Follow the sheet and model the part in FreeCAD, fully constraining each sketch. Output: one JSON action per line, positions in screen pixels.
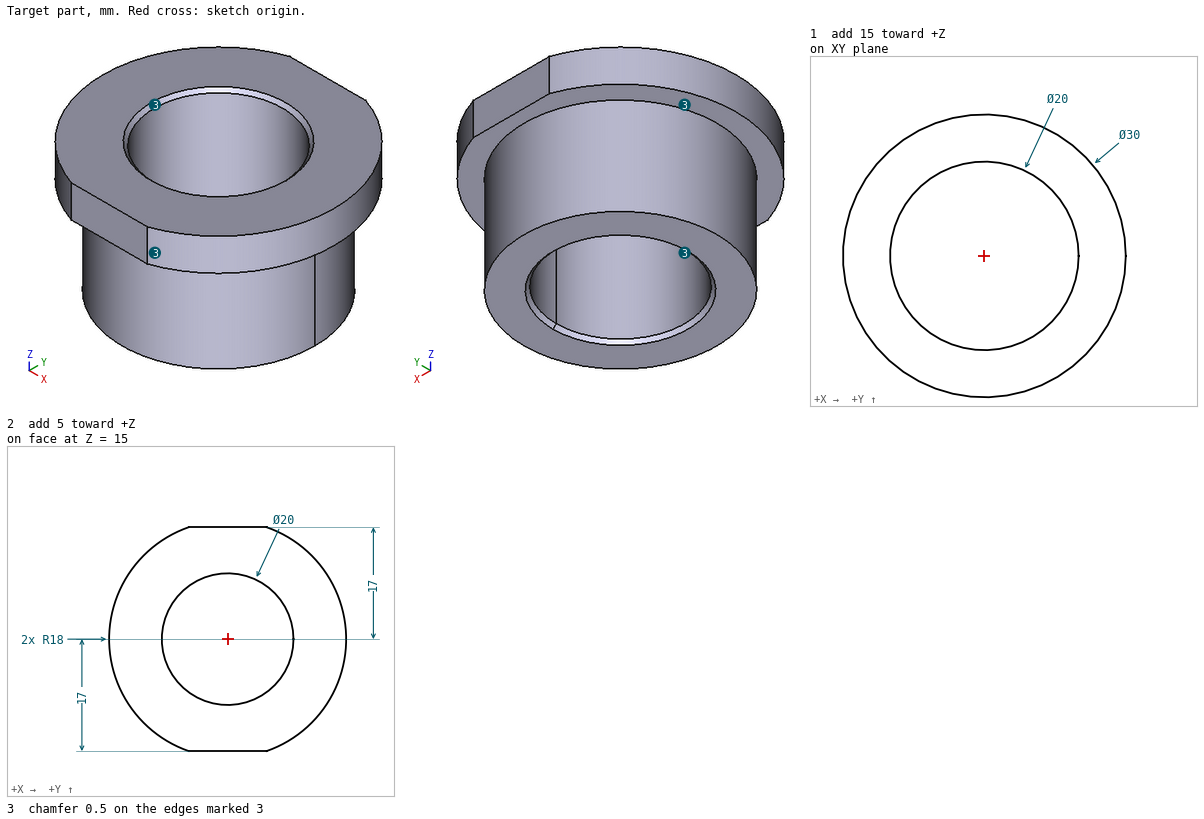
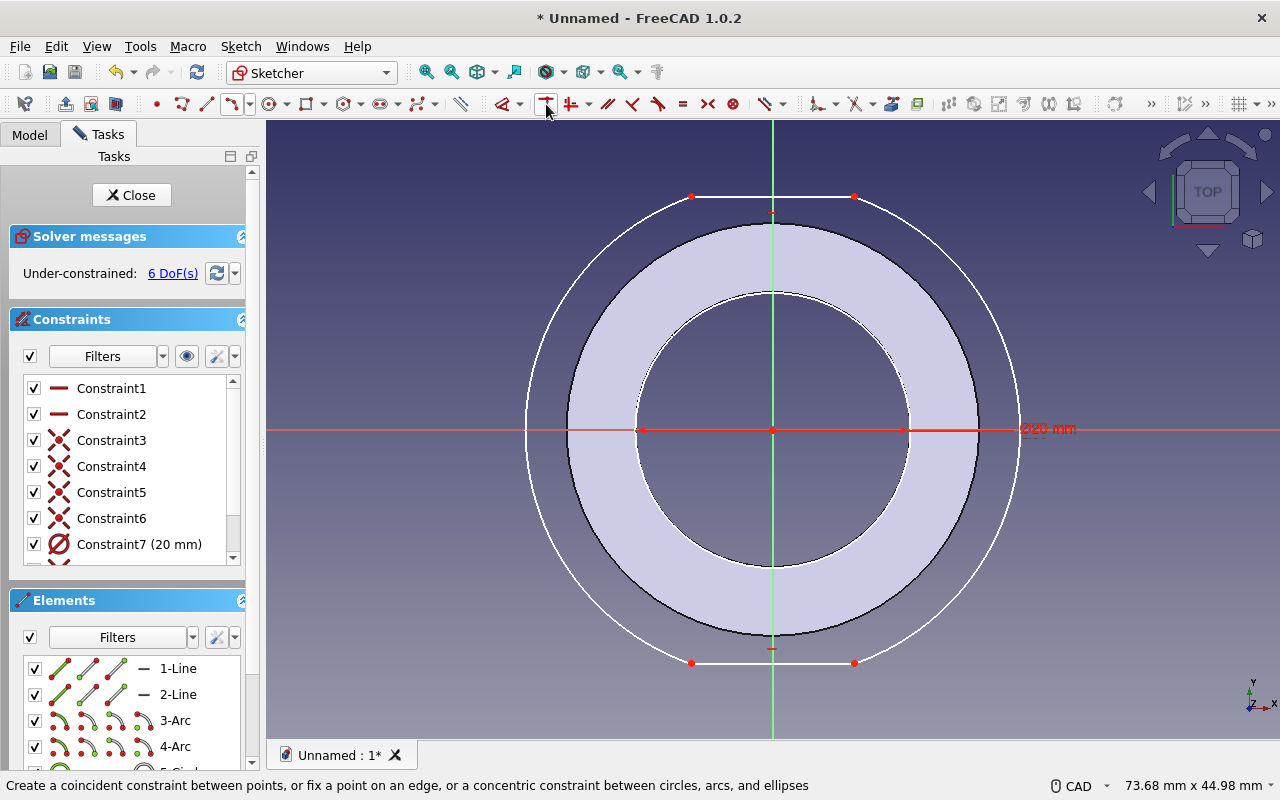
{"action": "left_click_drag", "start_coordinate": [763, 420], "coordinate": [783, 440]}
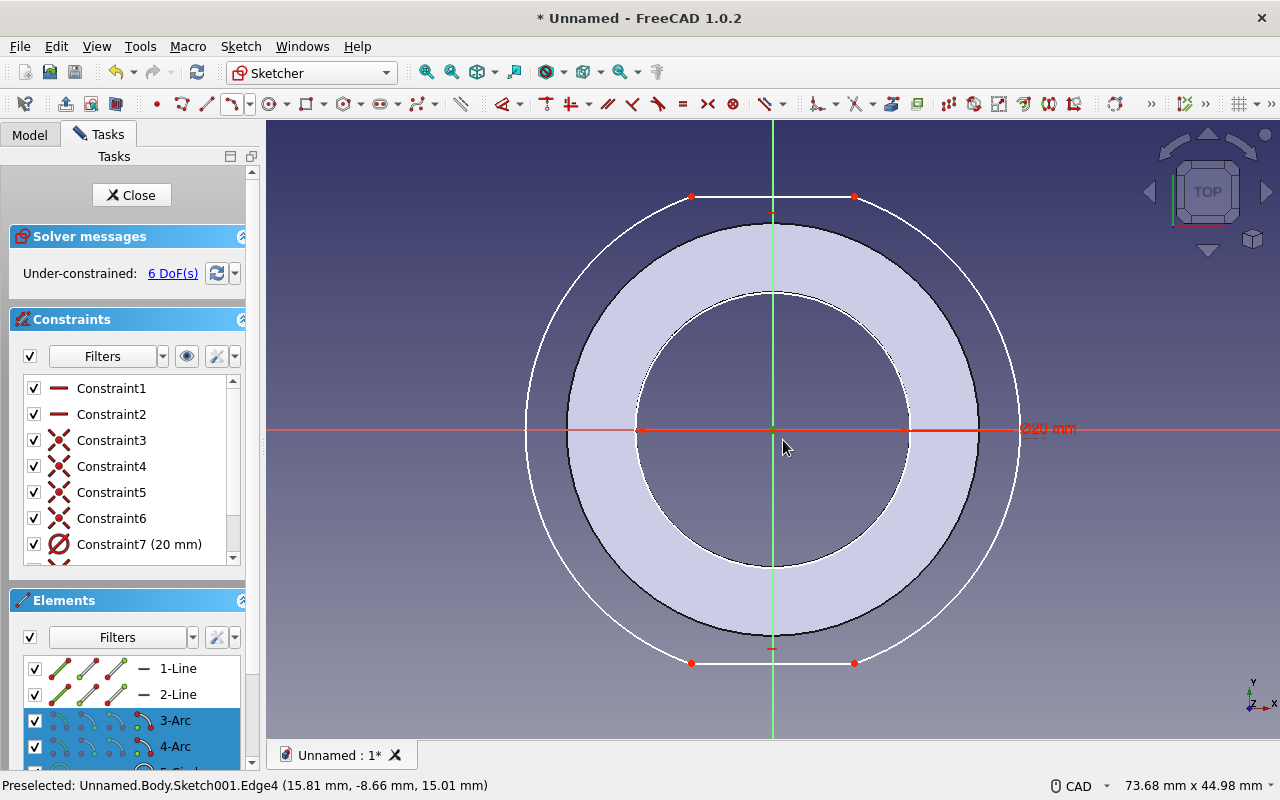
{"action": "left_click", "coordinate": [546, 104]}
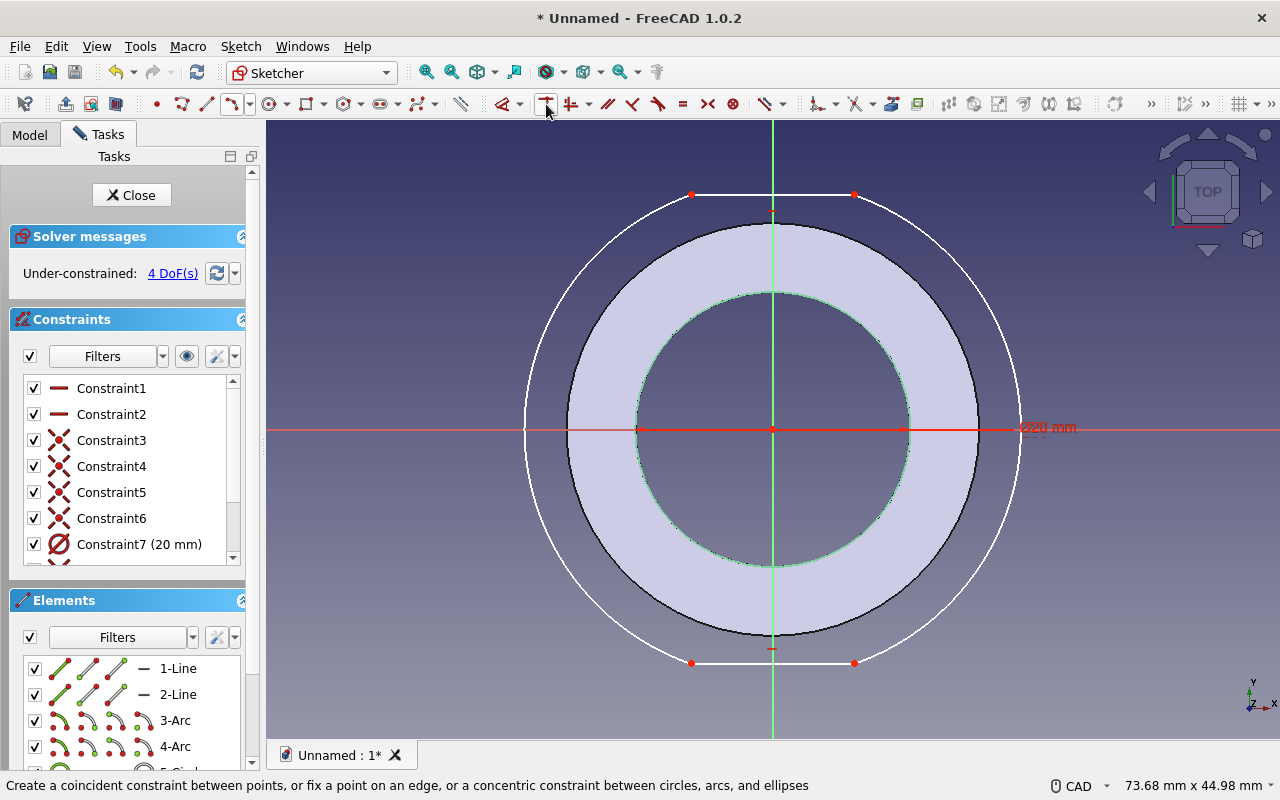
{"action": "left_click", "coordinate": [554, 312]}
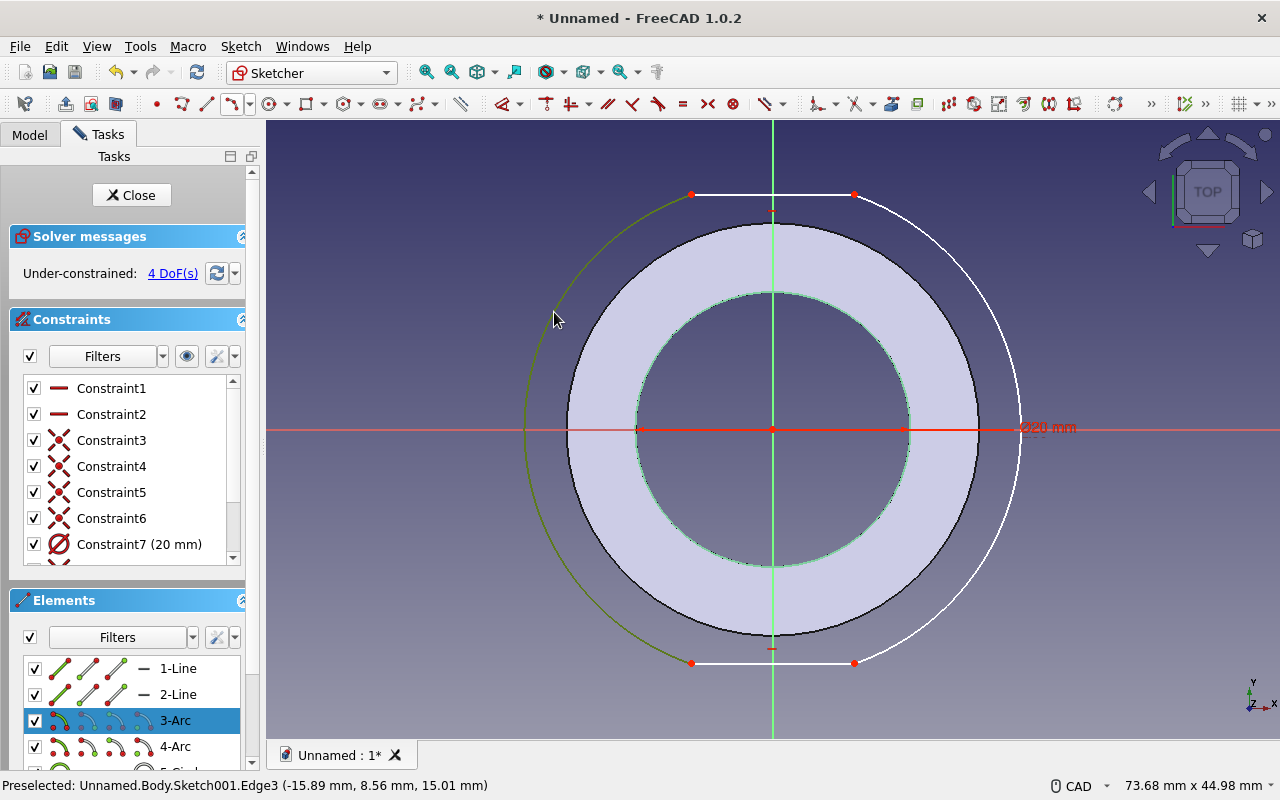
{"action": "left_click", "coordinate": [991, 547]}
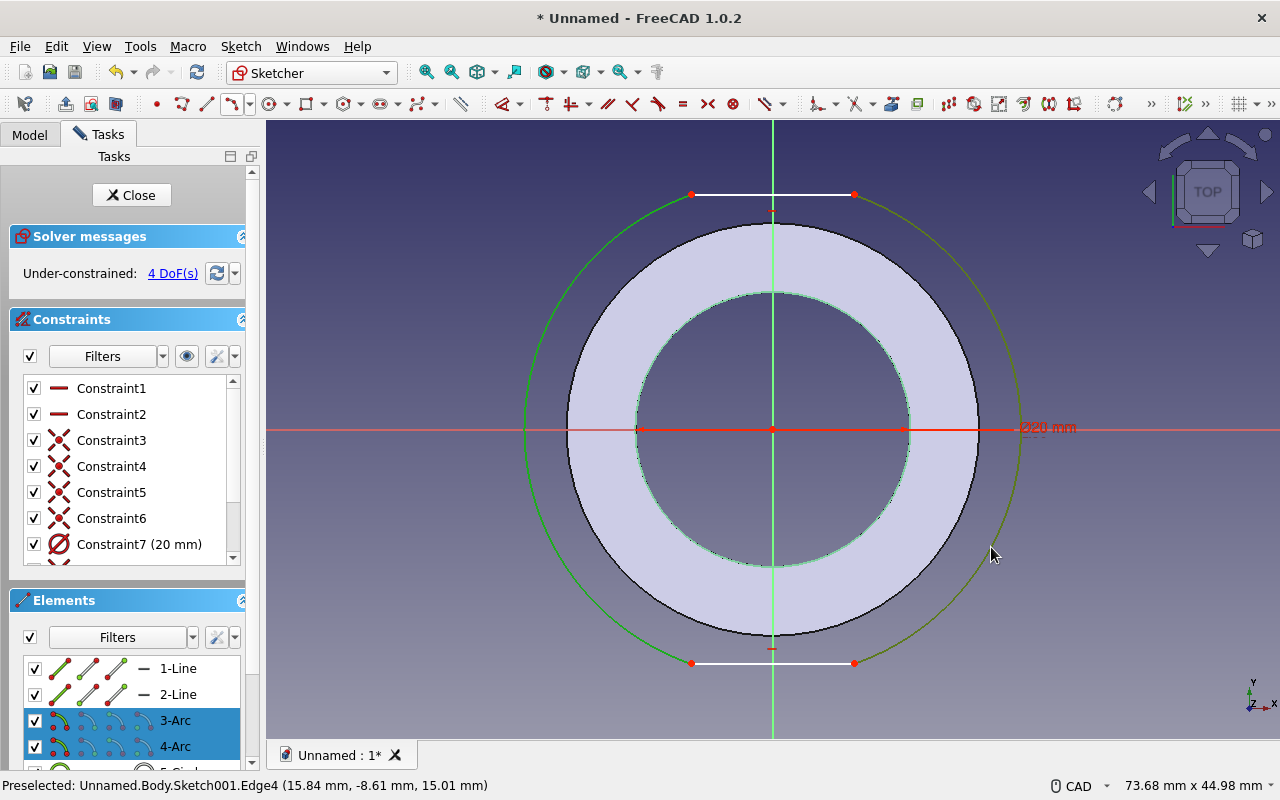
{"action": "left_click", "coordinate": [683, 104]}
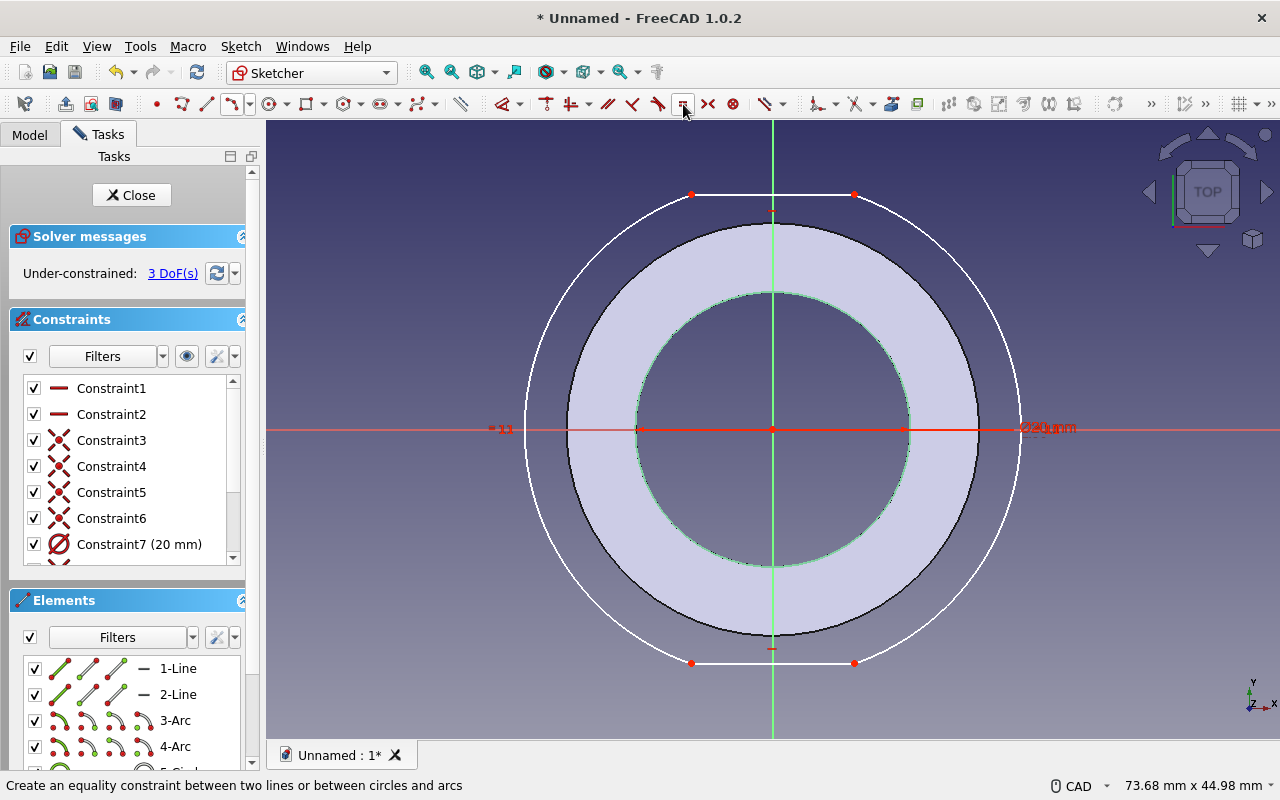
{"action": "left_click", "coordinate": [502, 104]}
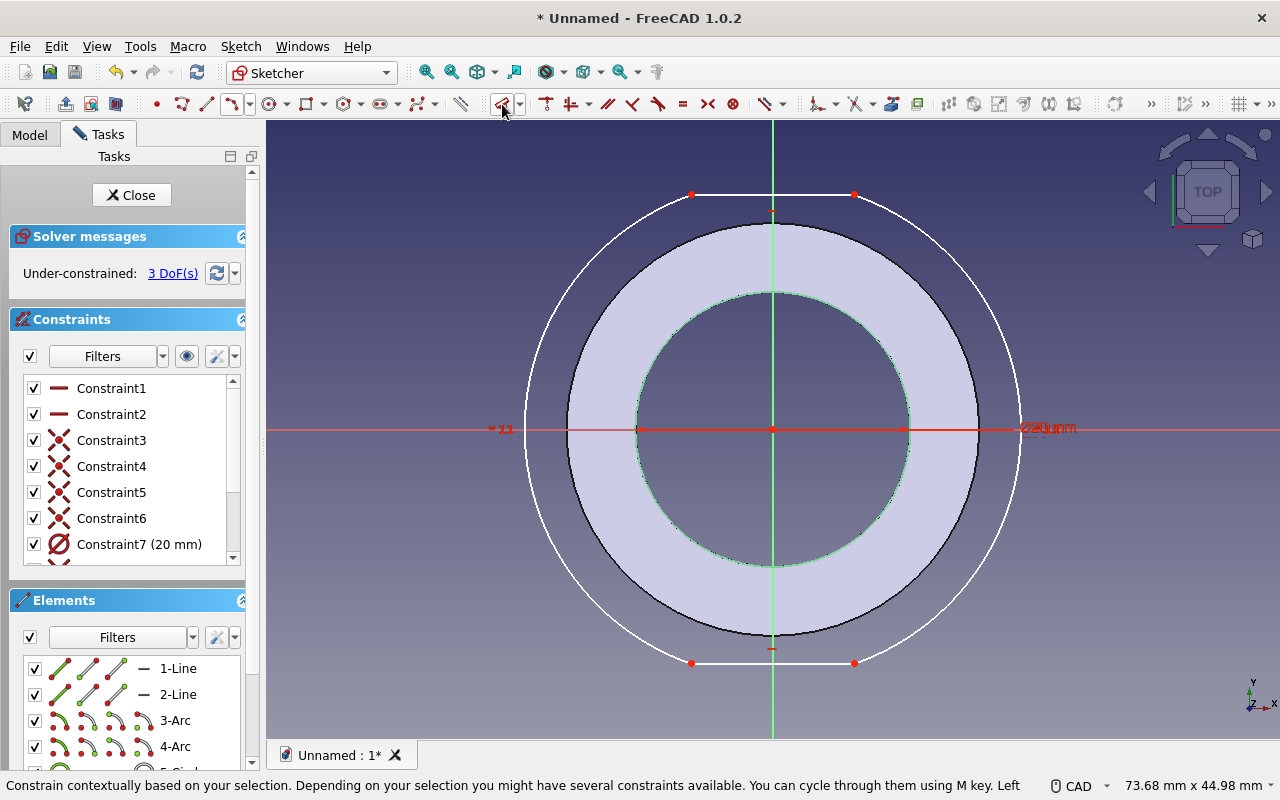
{"action": "left_click", "coordinate": [554, 312]}
{"action": "left_click", "coordinate": [526, 297]}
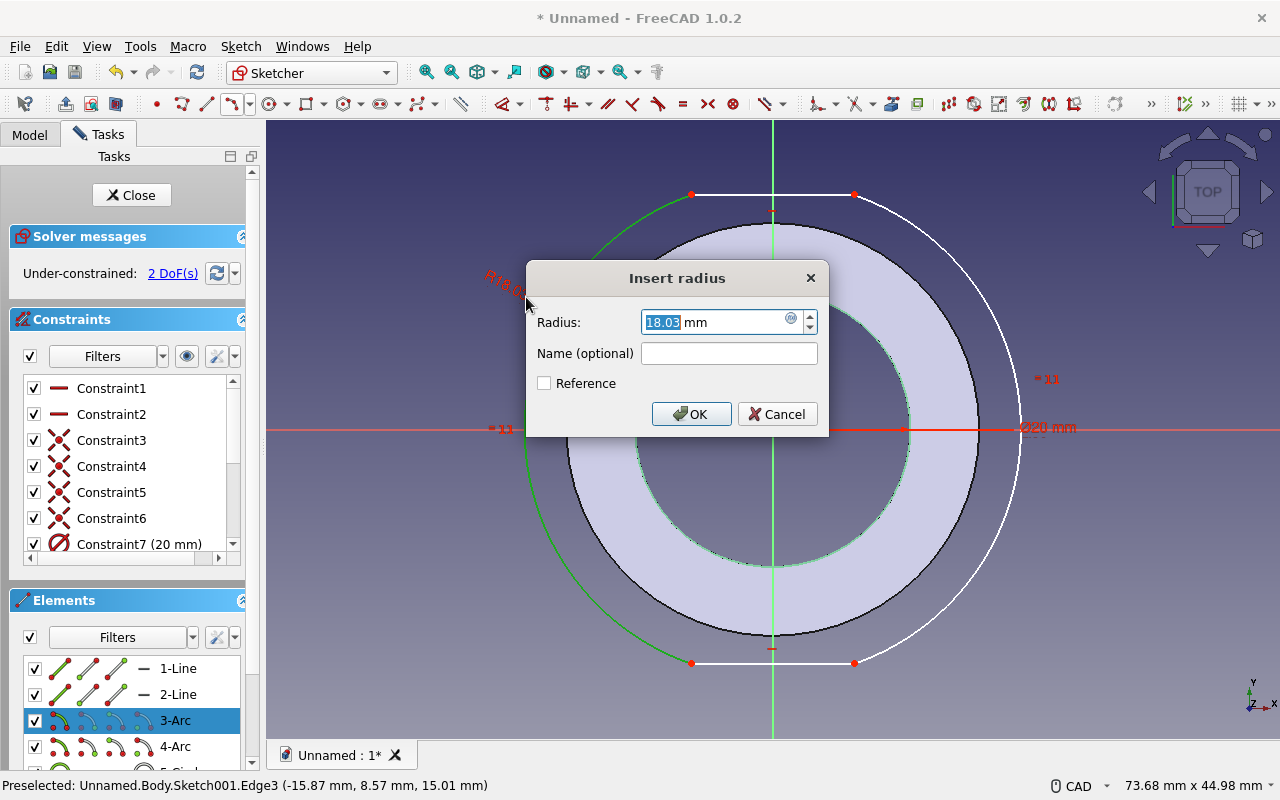
{"action": "type", "text": "18"}
{"action": "key", "text": "Return"}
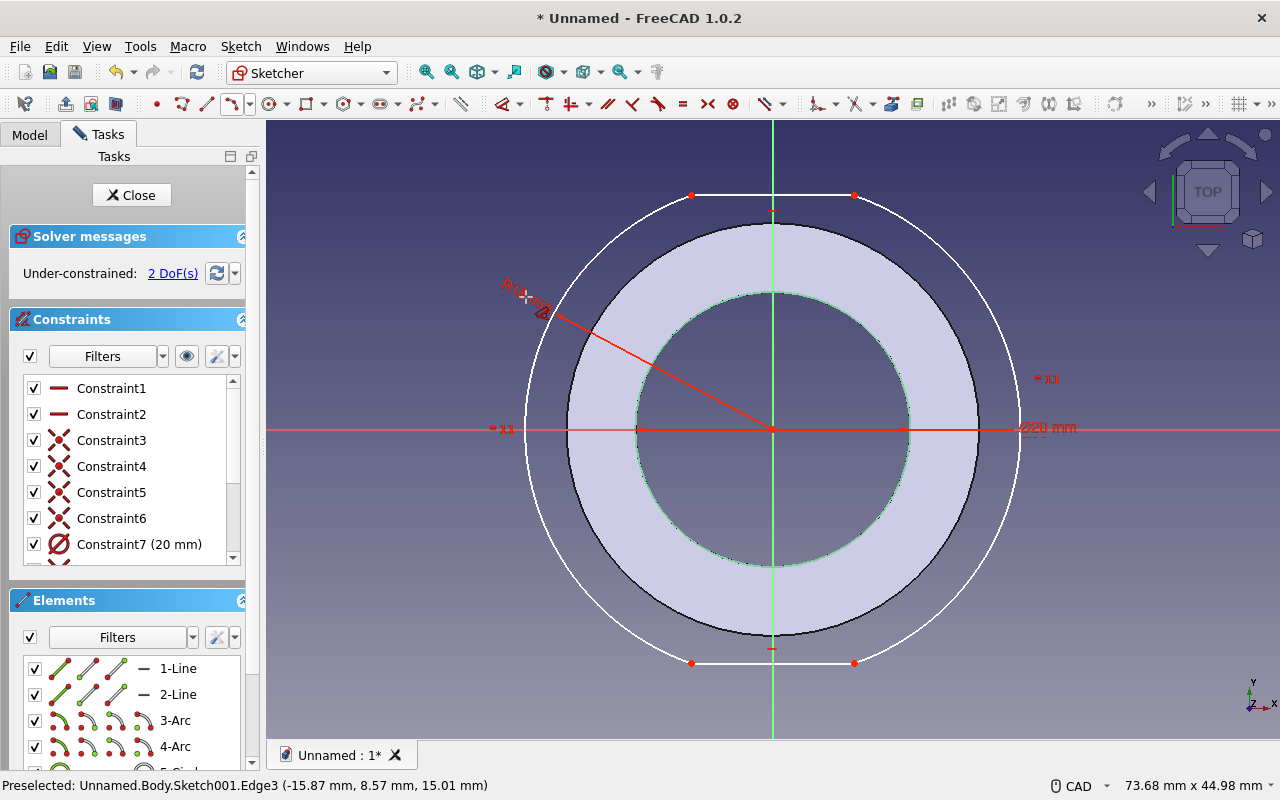
{"action": "left_click", "coordinate": [854, 195]}
{"action": "left_click", "coordinate": [888, 312]}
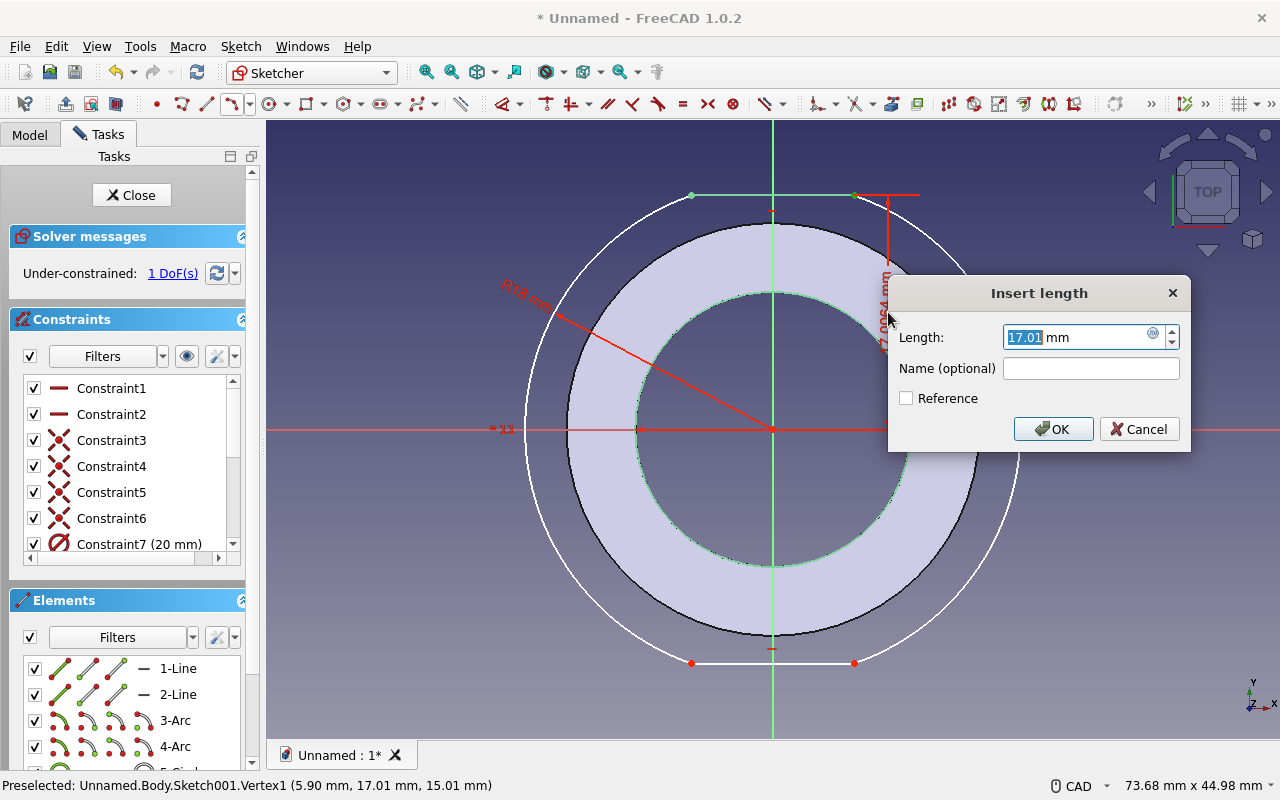
{"action": "type", "text": "17"}
{"action": "key", "text": "Return"}